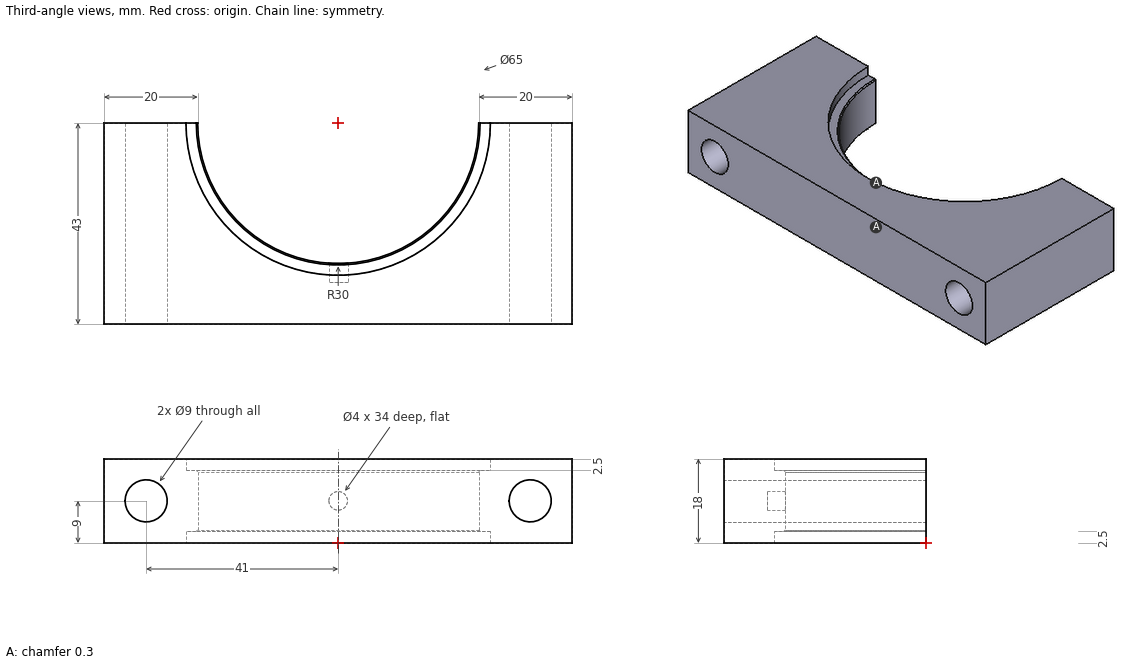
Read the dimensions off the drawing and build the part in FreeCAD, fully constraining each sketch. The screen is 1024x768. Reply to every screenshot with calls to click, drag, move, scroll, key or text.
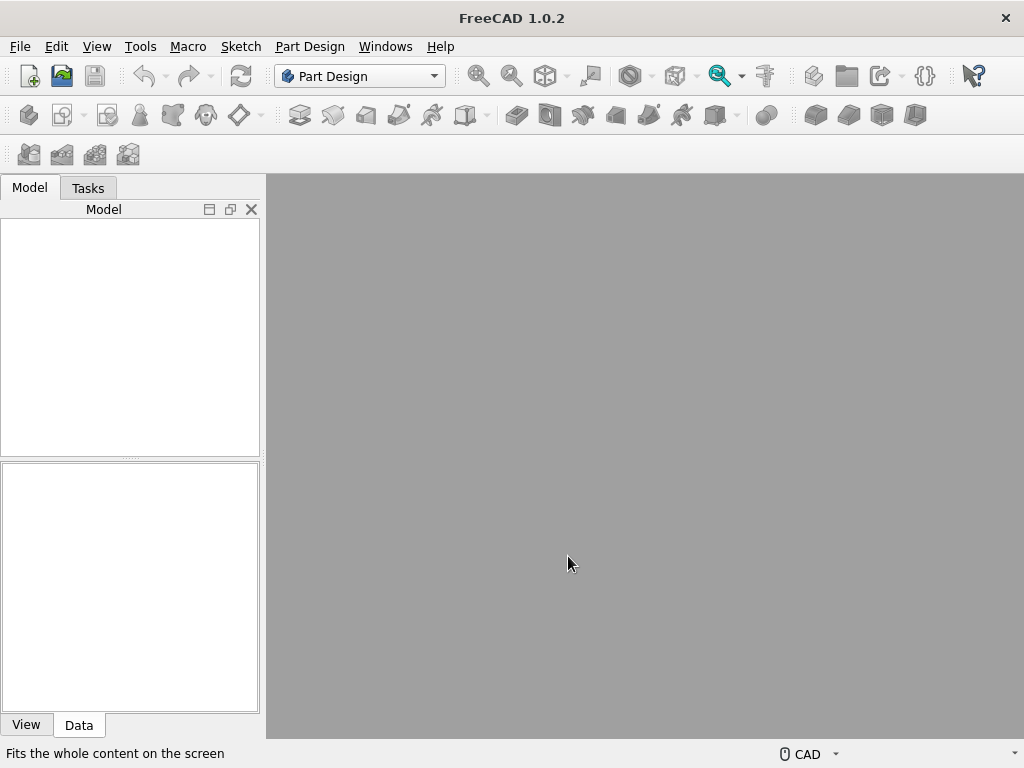
click(29, 76)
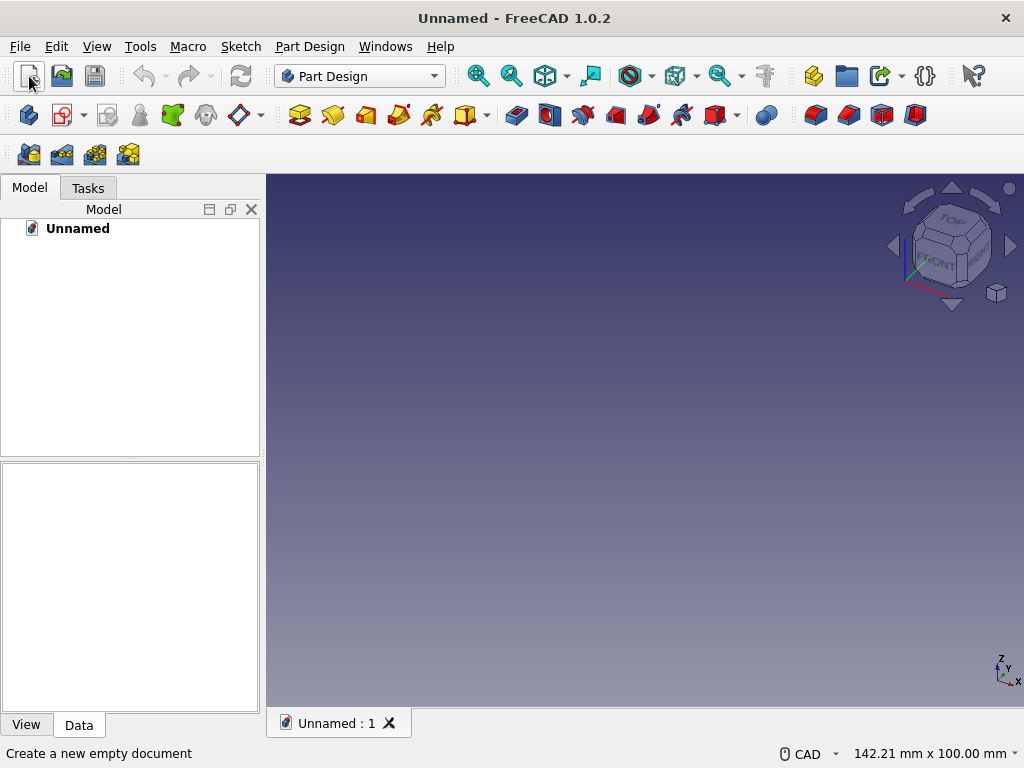
click(62, 116)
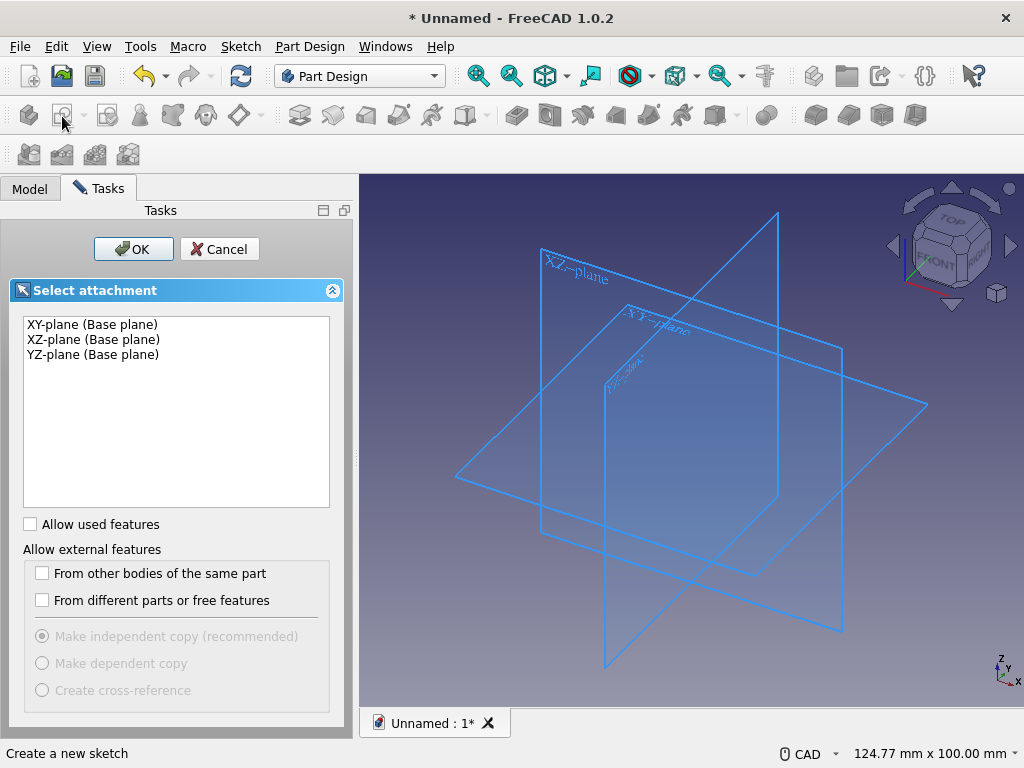
click(84, 324)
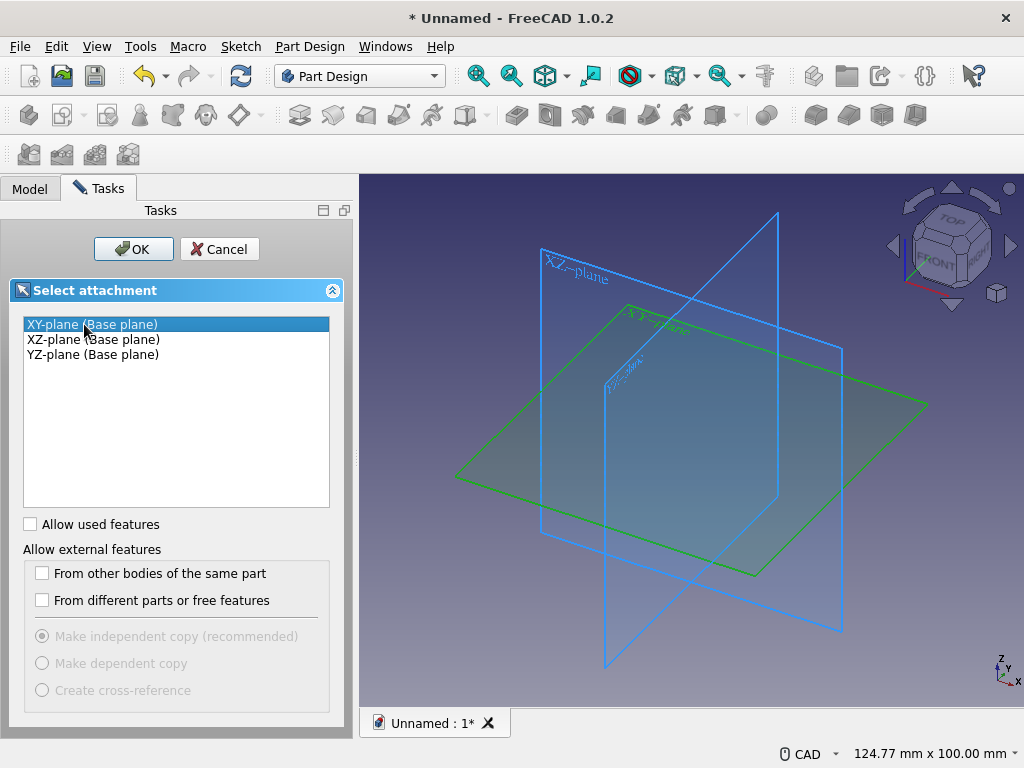
click(134, 249)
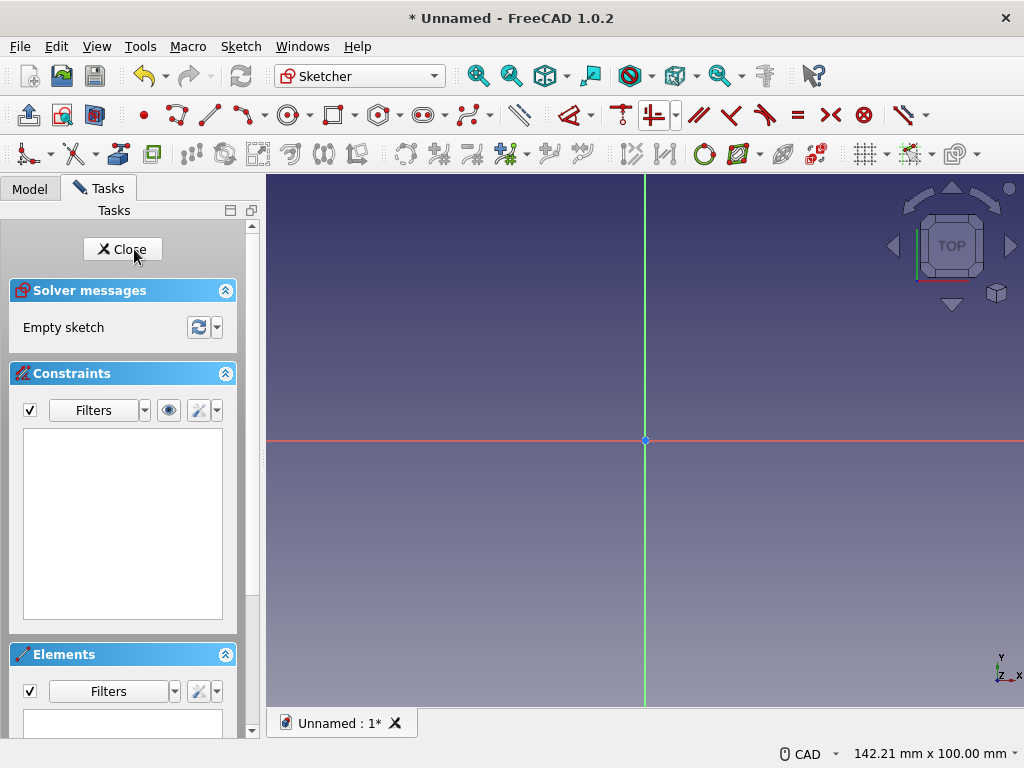
scroll(294, 202, down, 1)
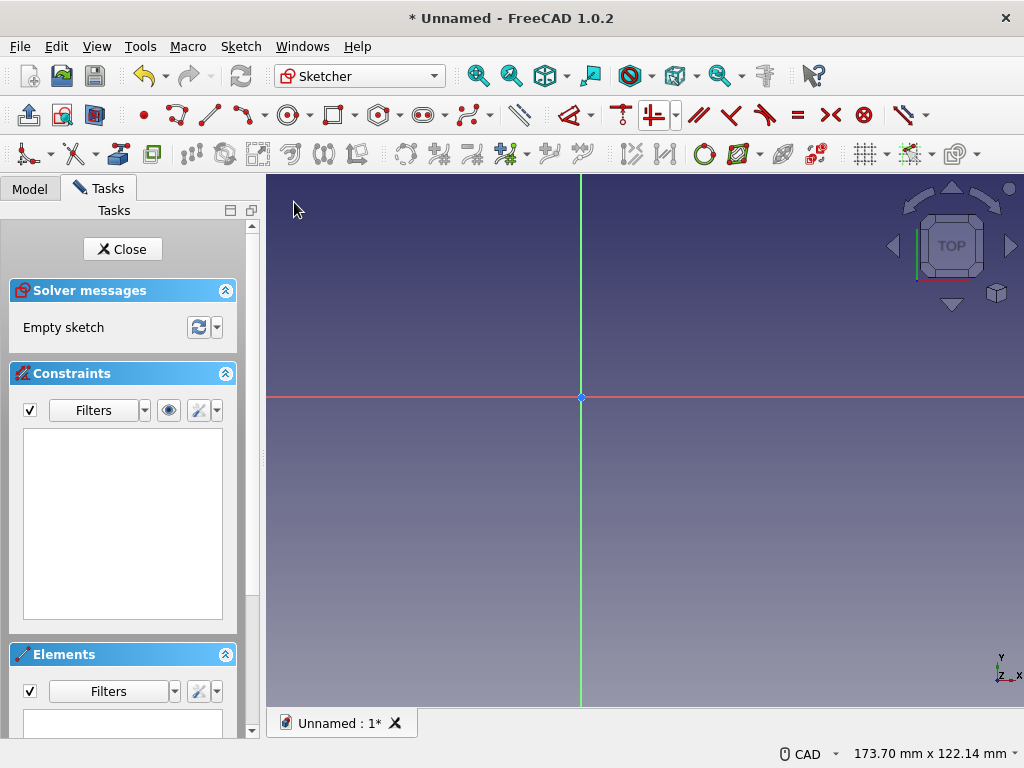
click(177, 116)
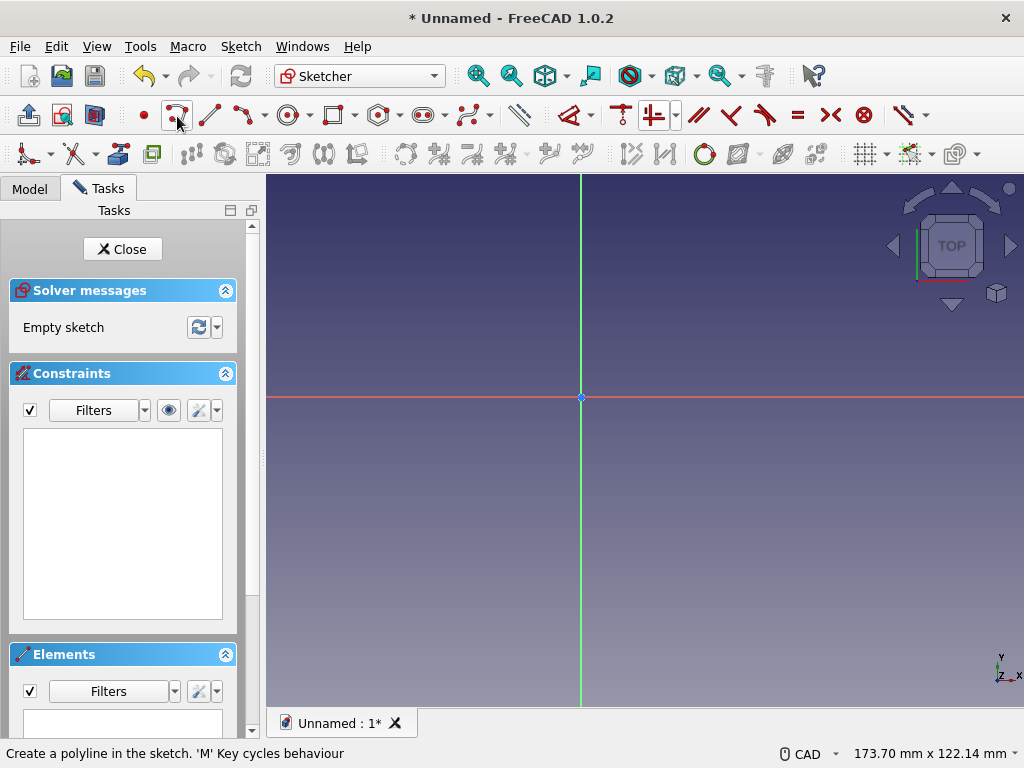
click(450, 397)
click(363, 406)
click(363, 585)
click(800, 585)
click(800, 397)
click(712, 406)
right_click(712, 406)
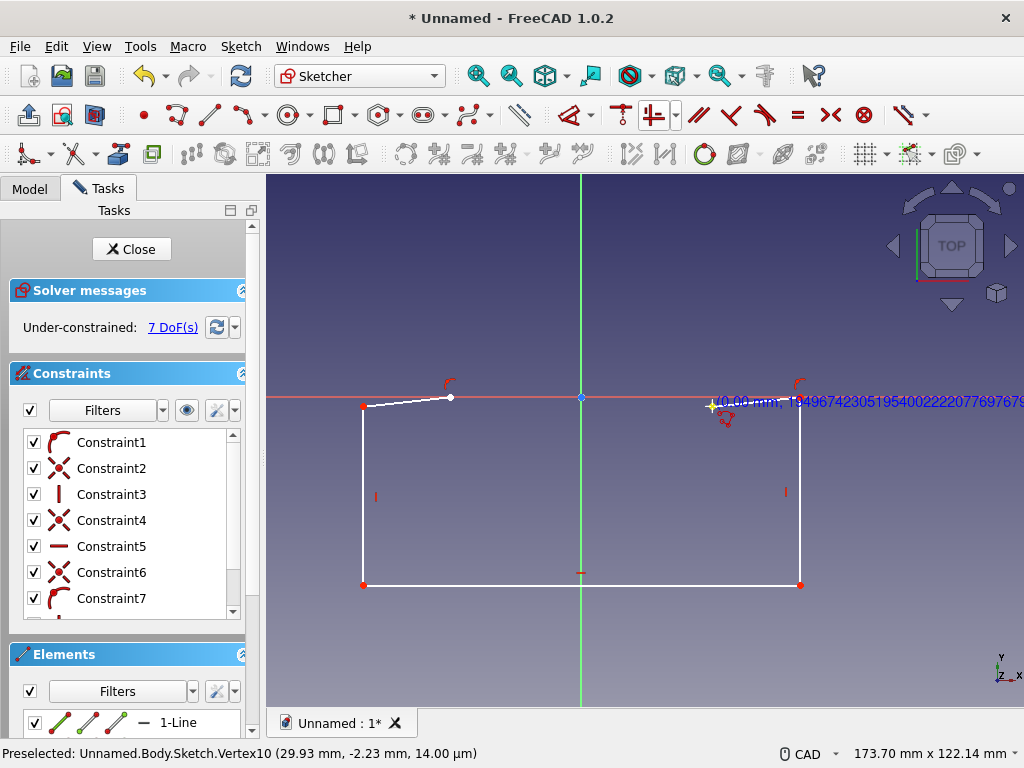
click(242, 116)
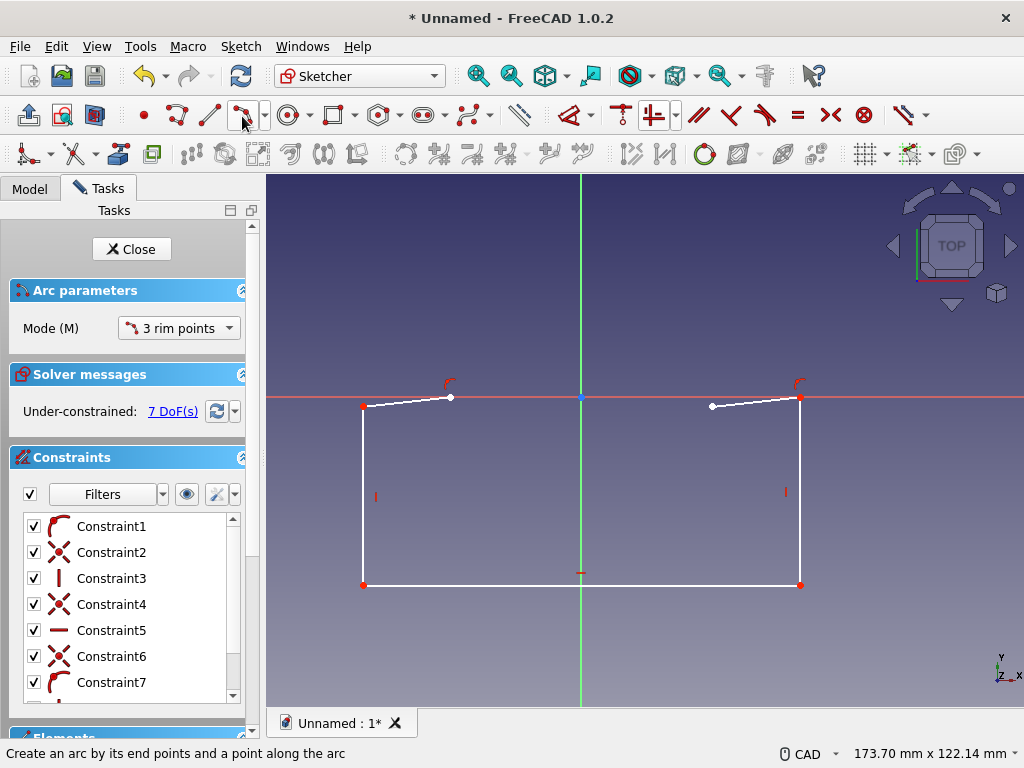
click(712, 407)
click(450, 397)
click(541, 522)
key(Escape)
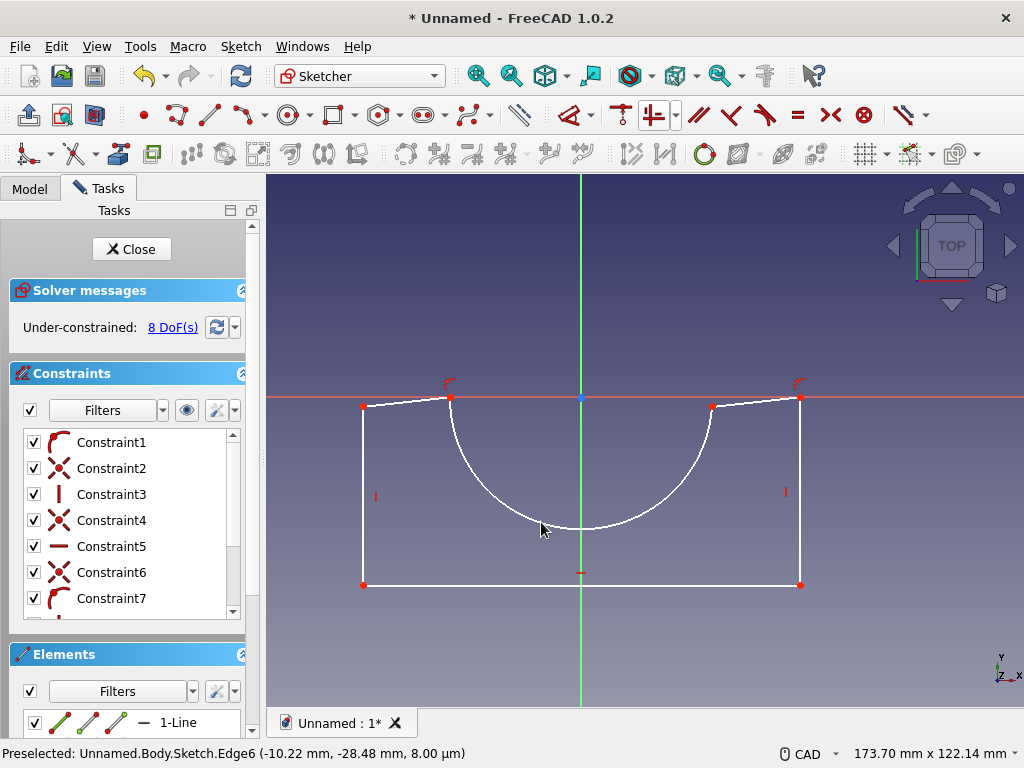
click(424, 400)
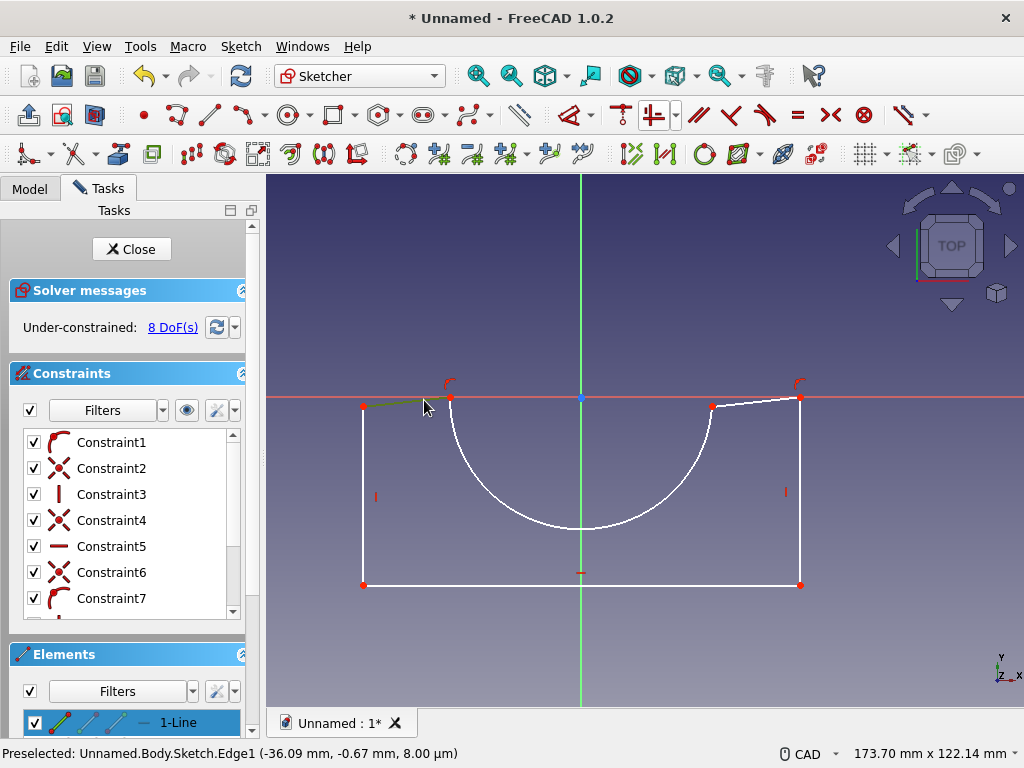
click(676, 116)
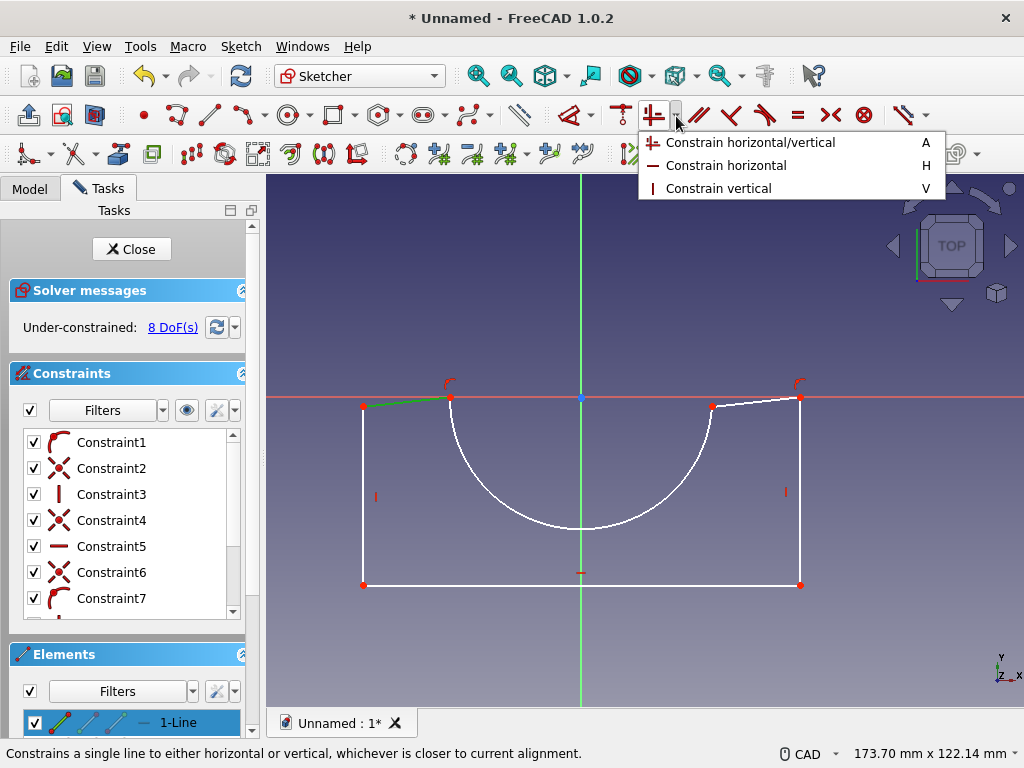
click(792, 166)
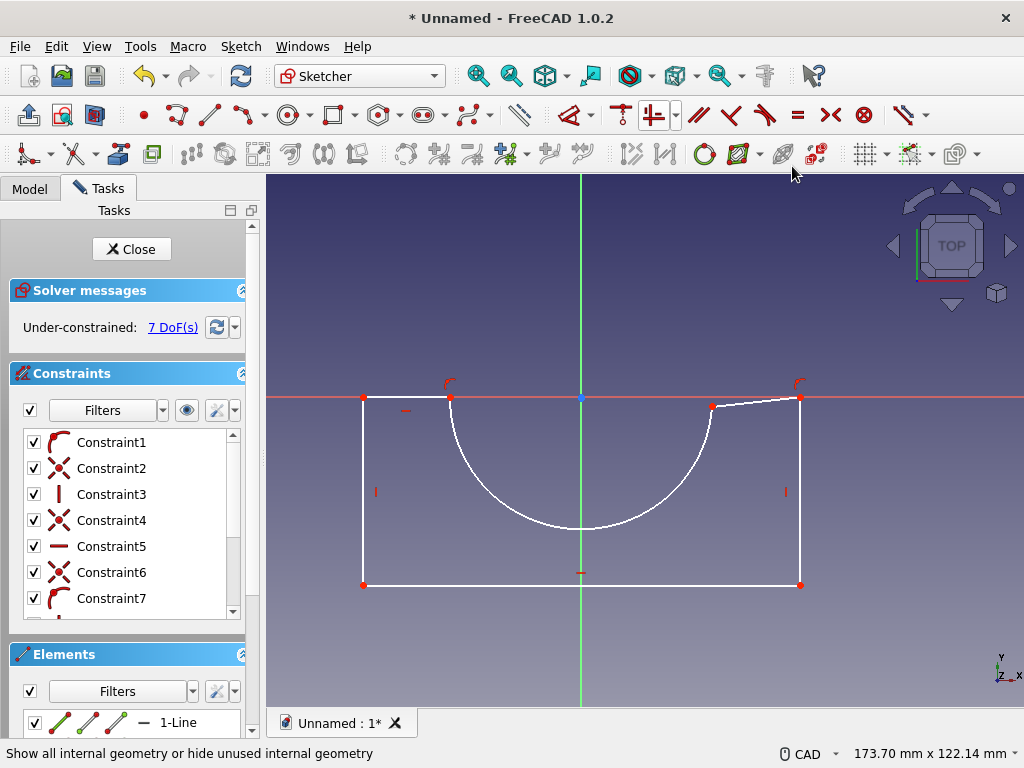
click(774, 400)